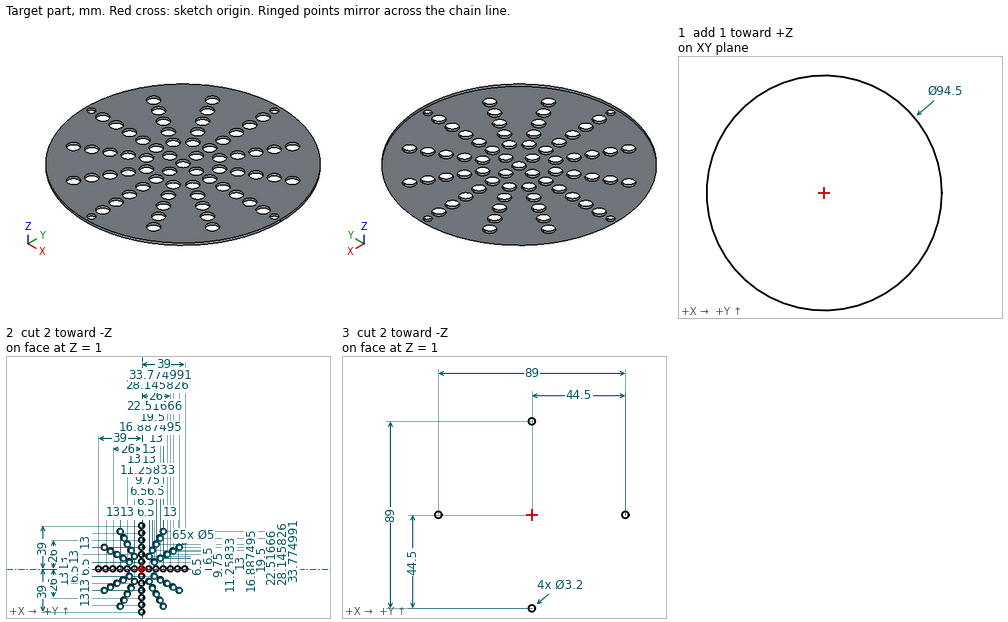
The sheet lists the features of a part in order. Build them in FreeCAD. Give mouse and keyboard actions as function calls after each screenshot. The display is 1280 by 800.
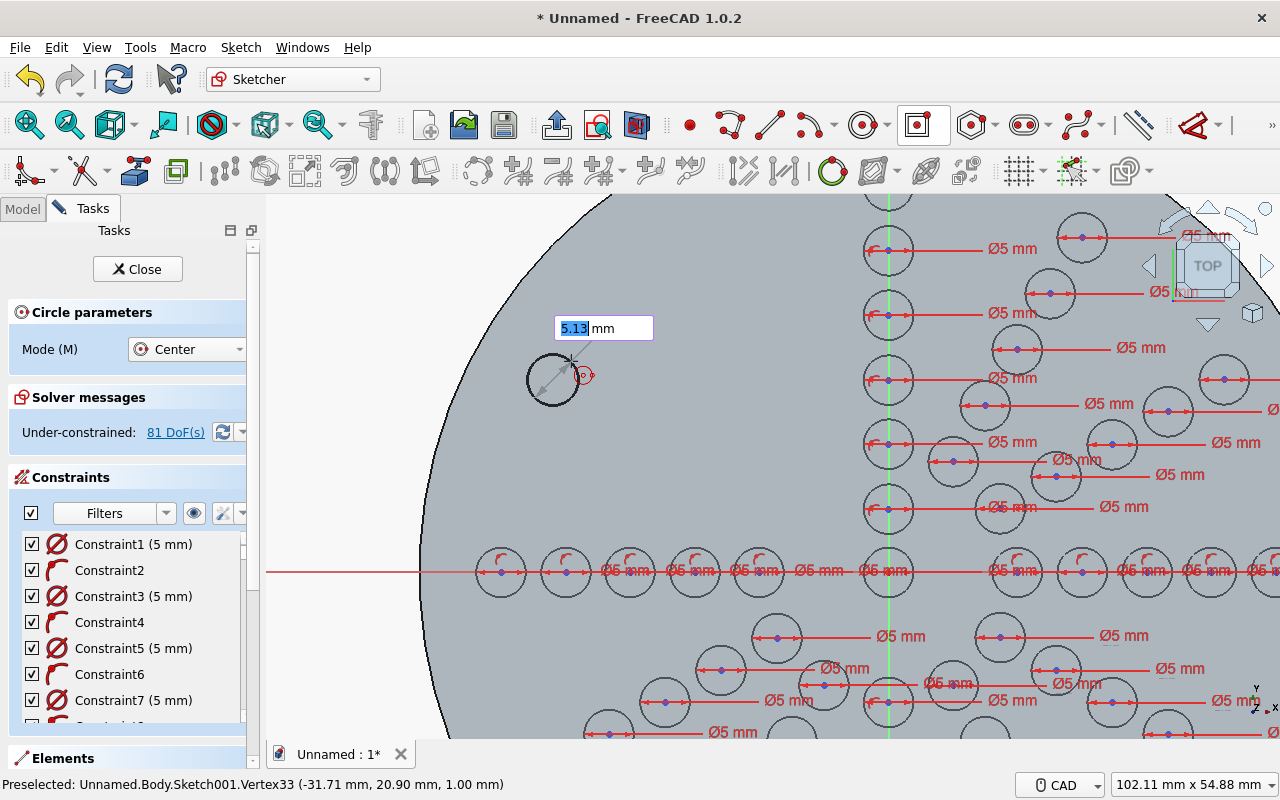
text(5)
key(Return)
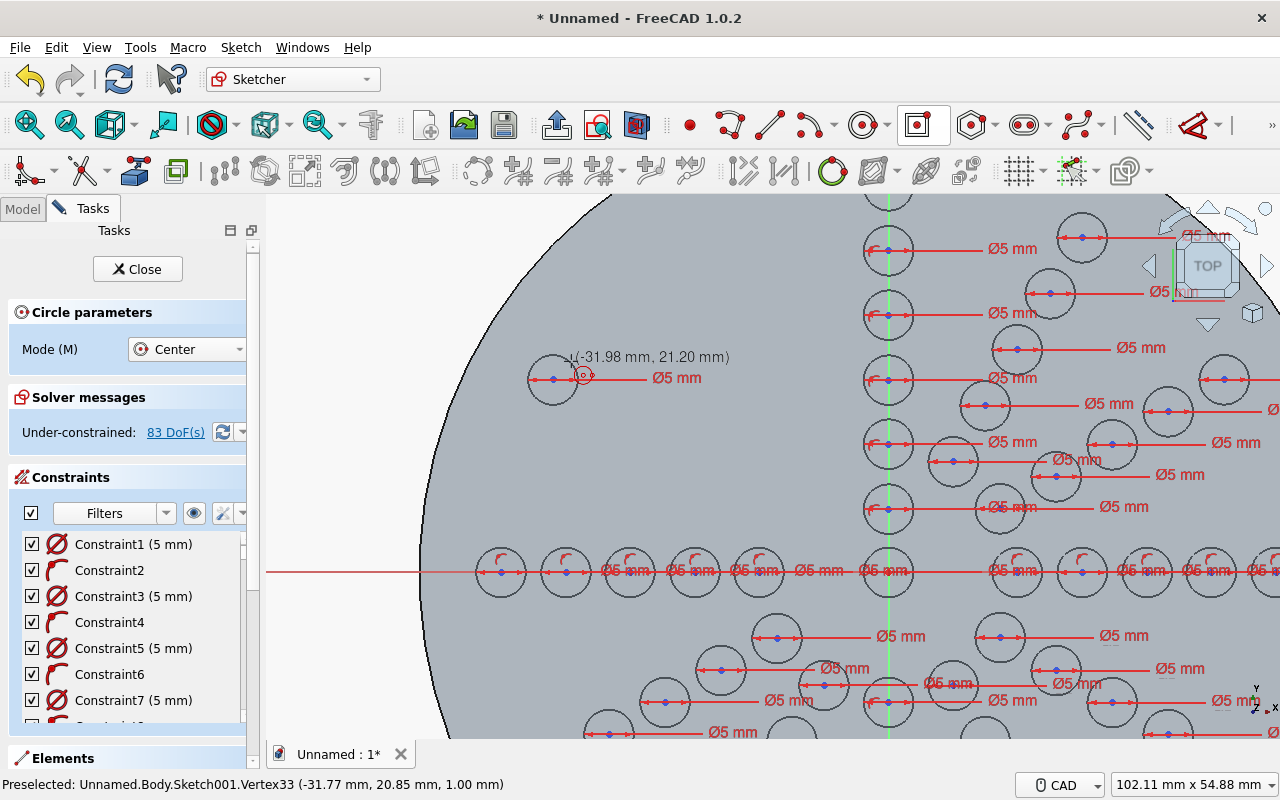
click(609, 411)
move(627, 394)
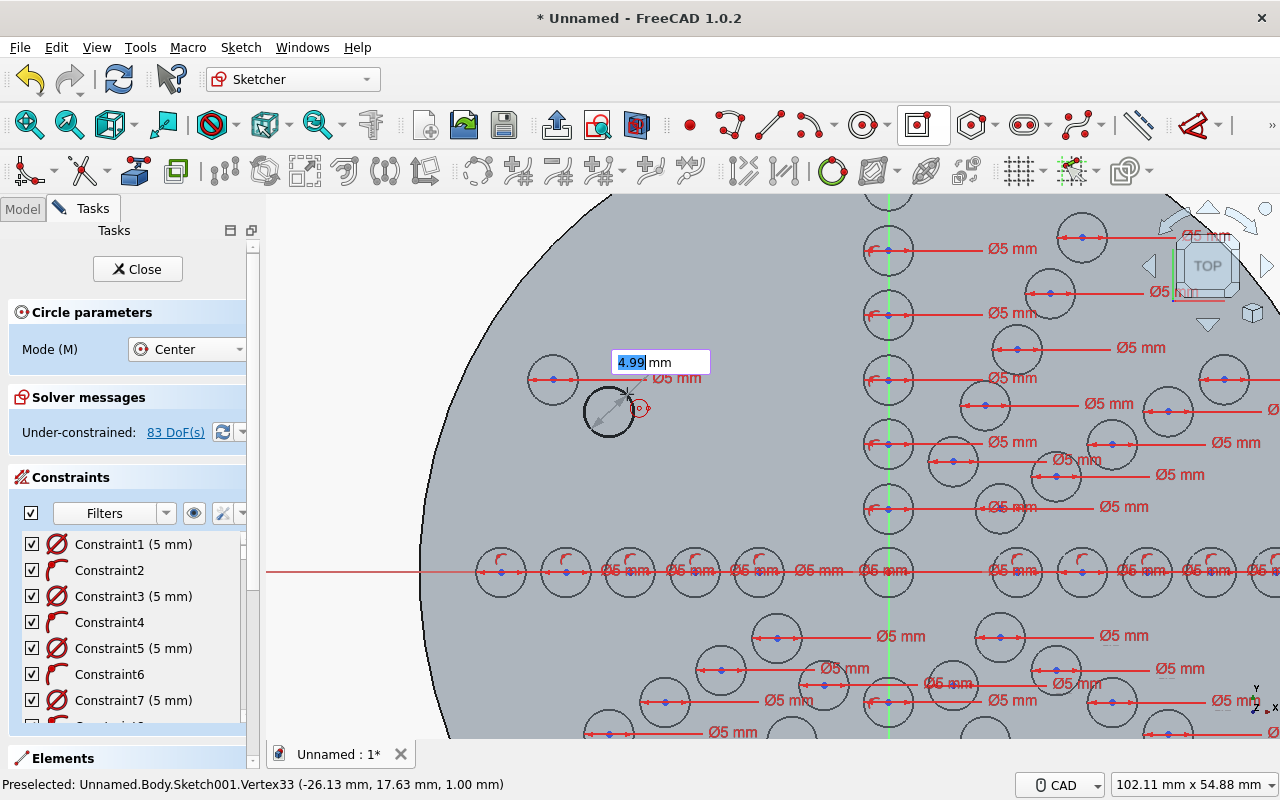
text(5)
key(Return)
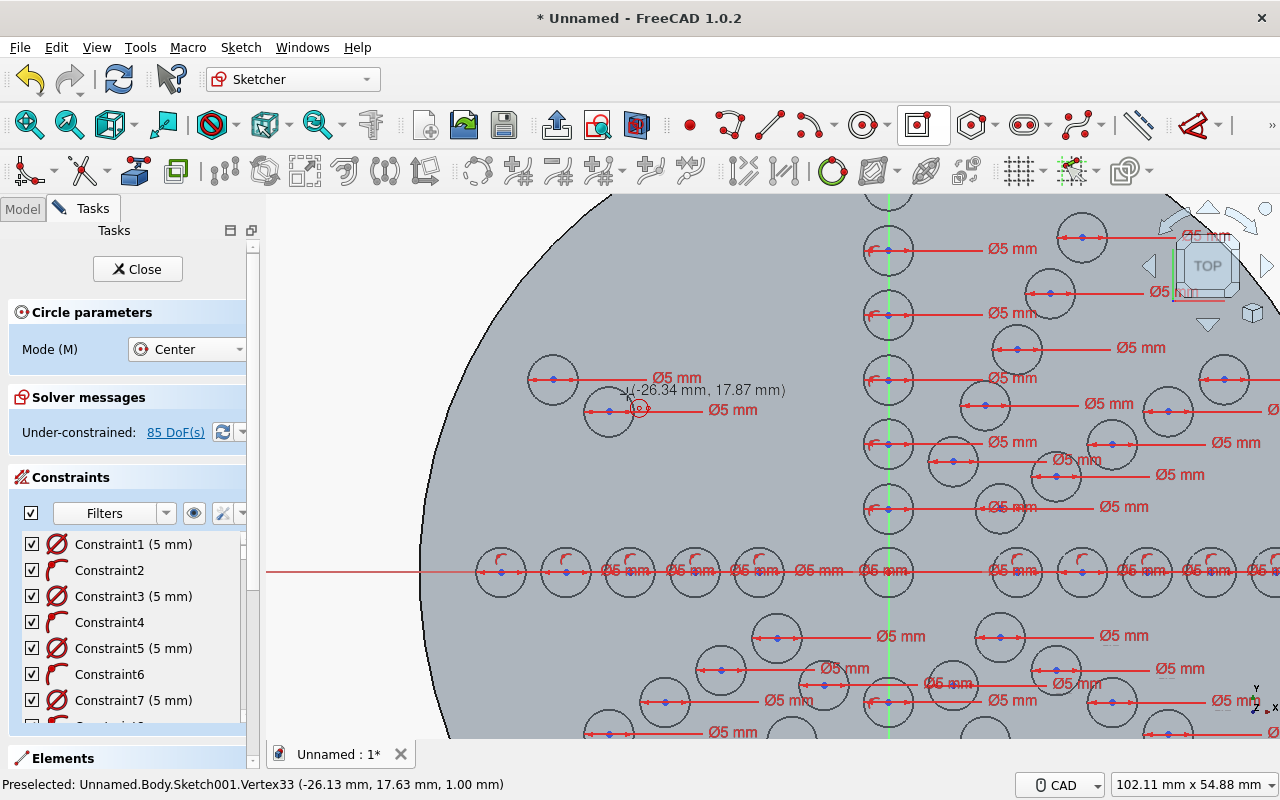
click(665, 443)
move(683, 426)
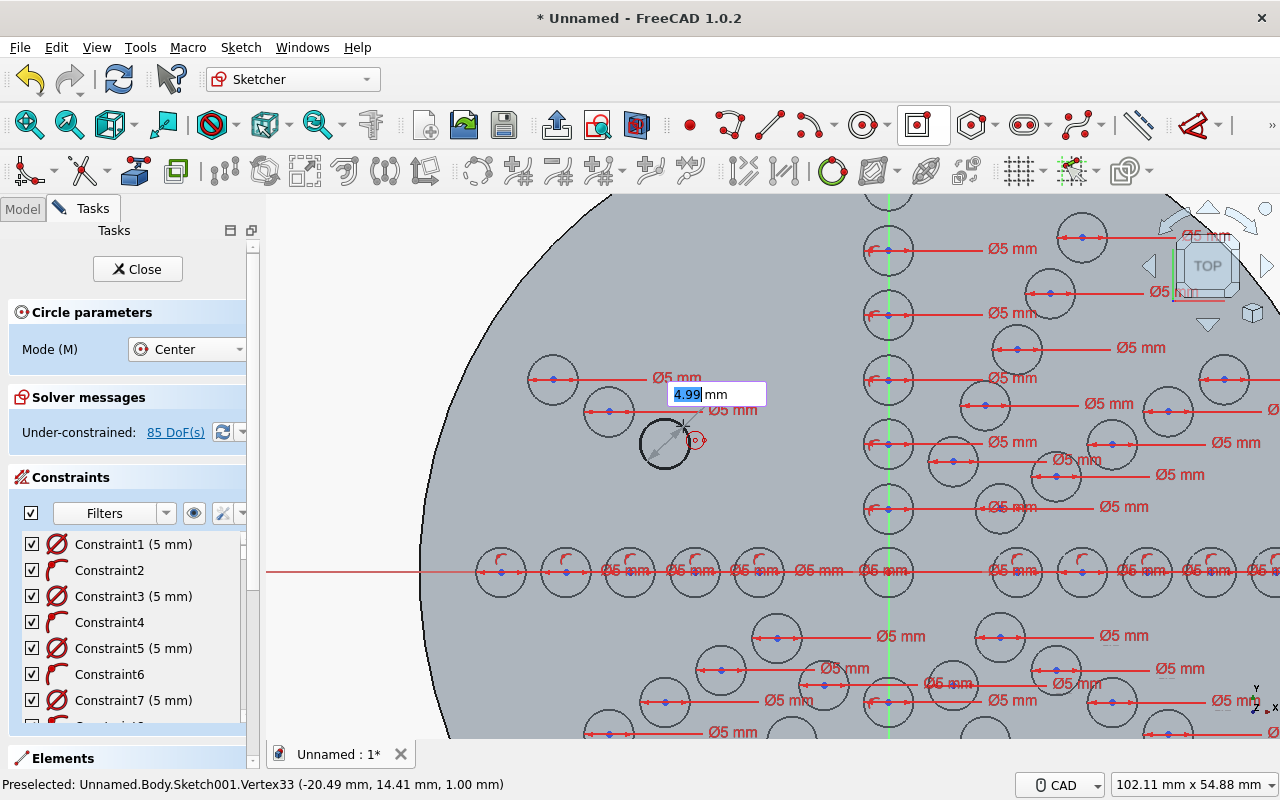
text(5)
key(Return)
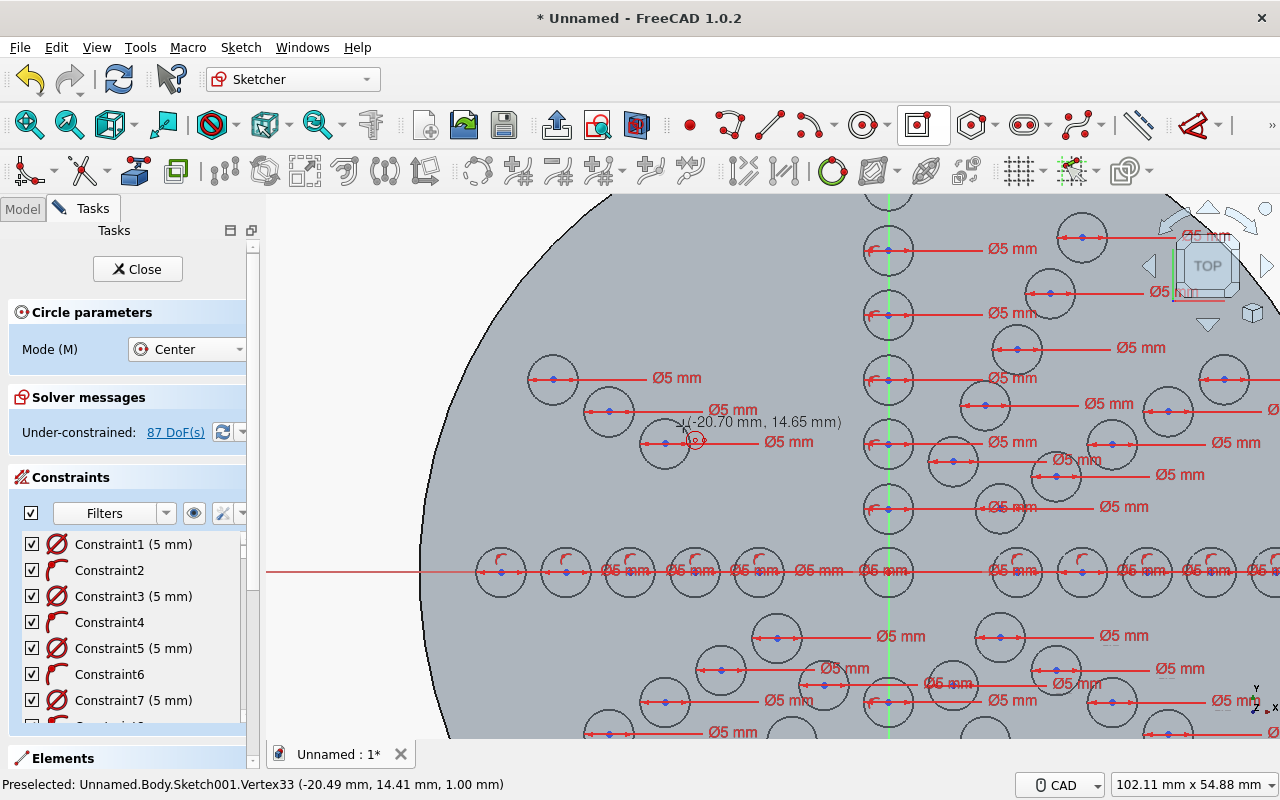
click(721, 476)
move(738, 458)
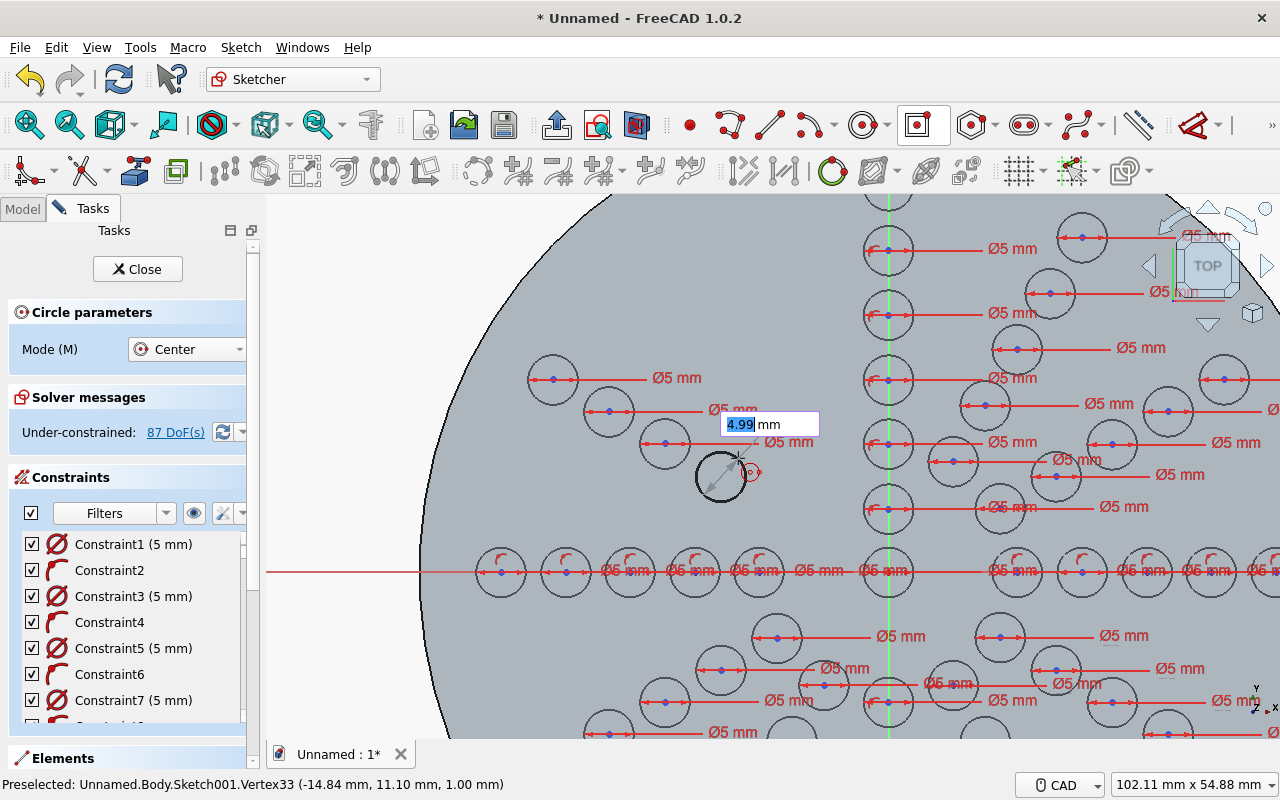
text(5)
key(Return)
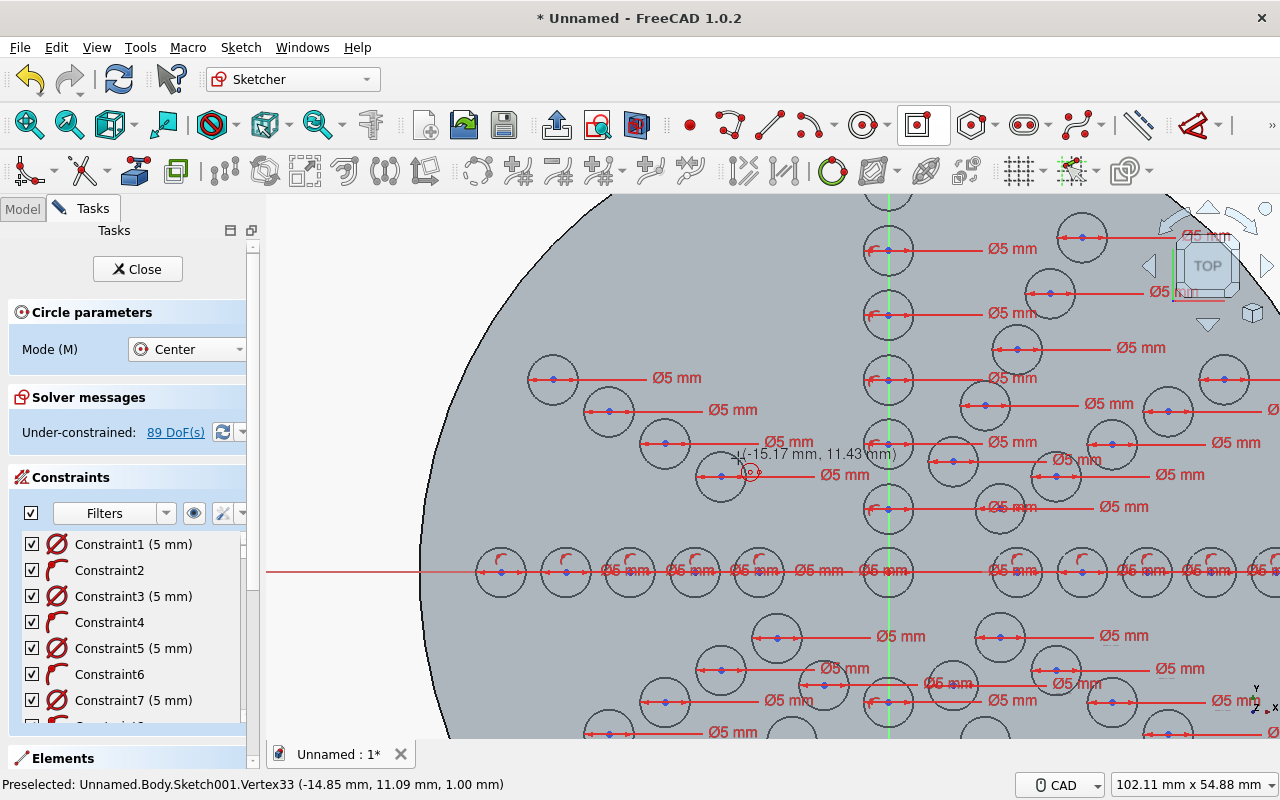
click(777, 508)
move(794, 490)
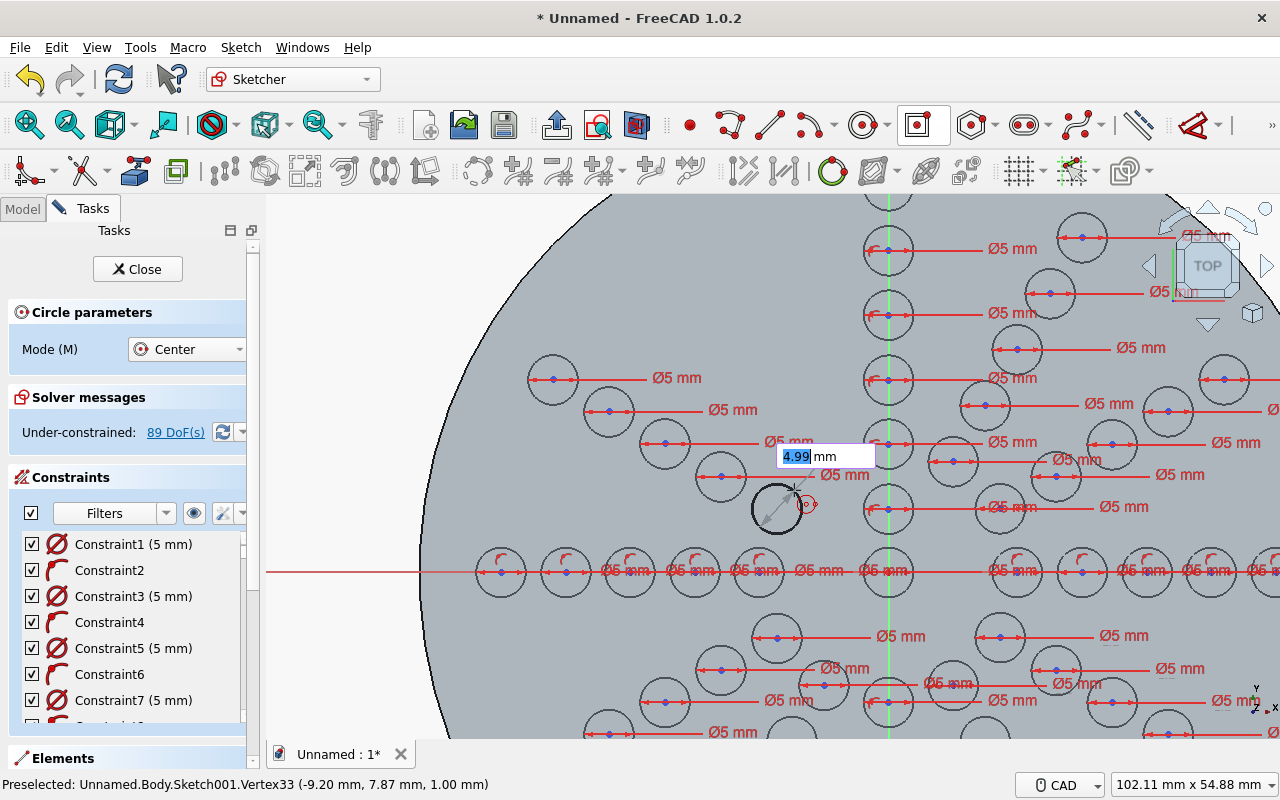
text(5)
key(Return)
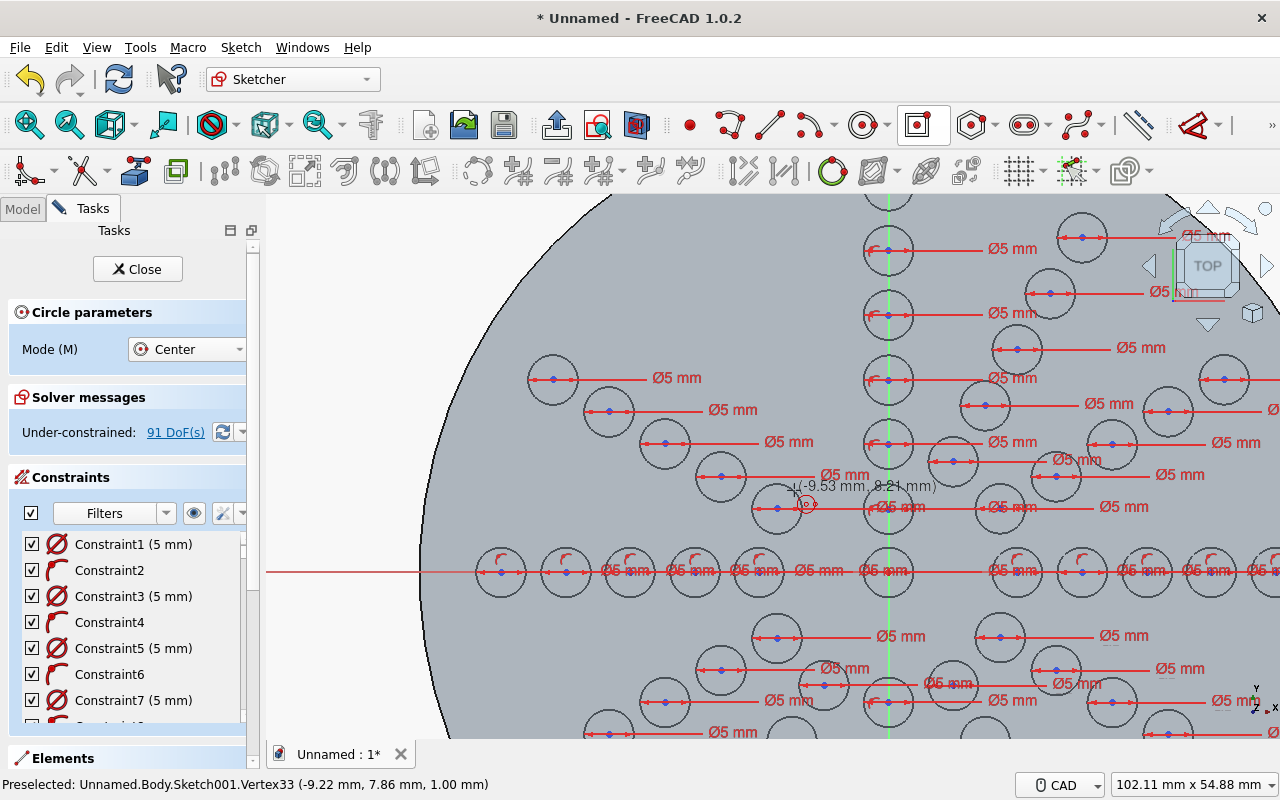
click(695, 237)